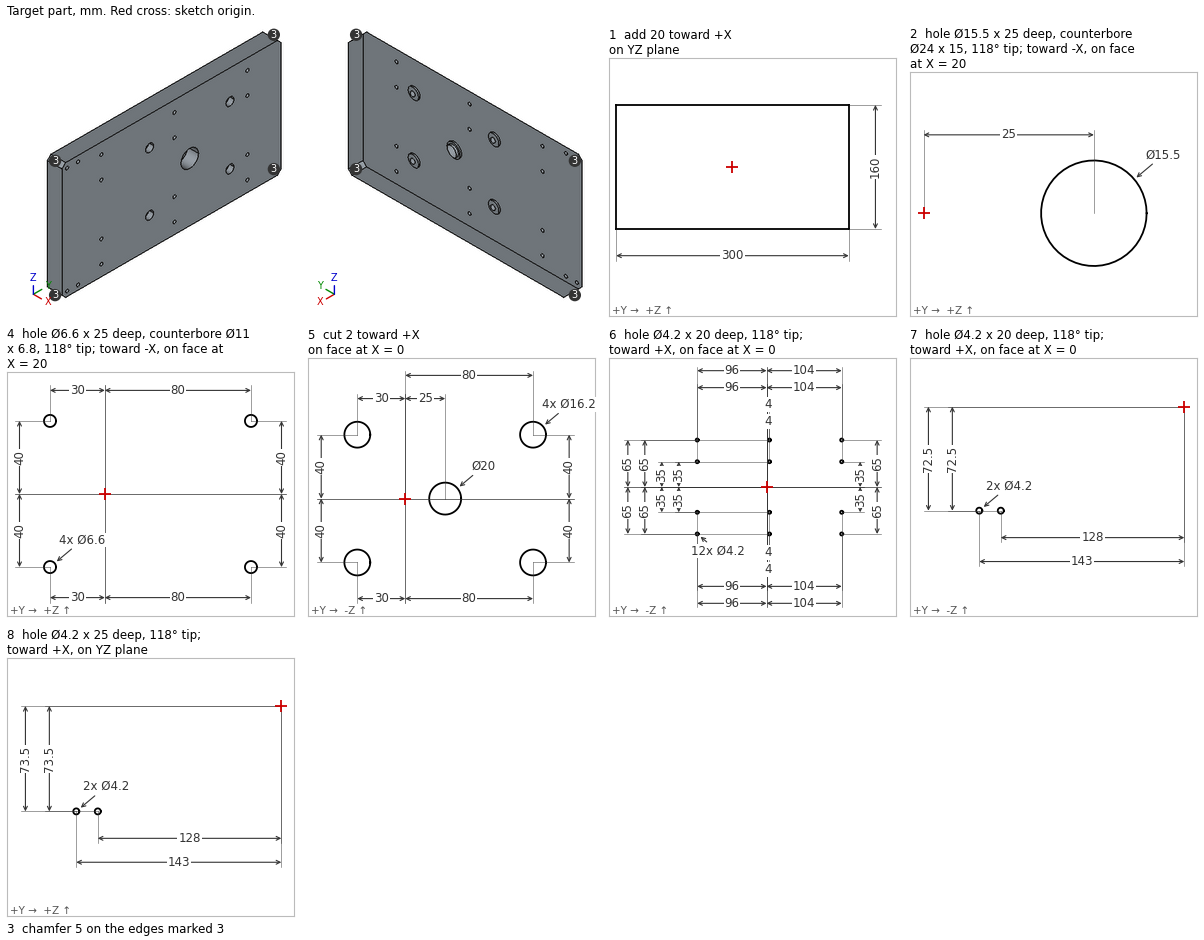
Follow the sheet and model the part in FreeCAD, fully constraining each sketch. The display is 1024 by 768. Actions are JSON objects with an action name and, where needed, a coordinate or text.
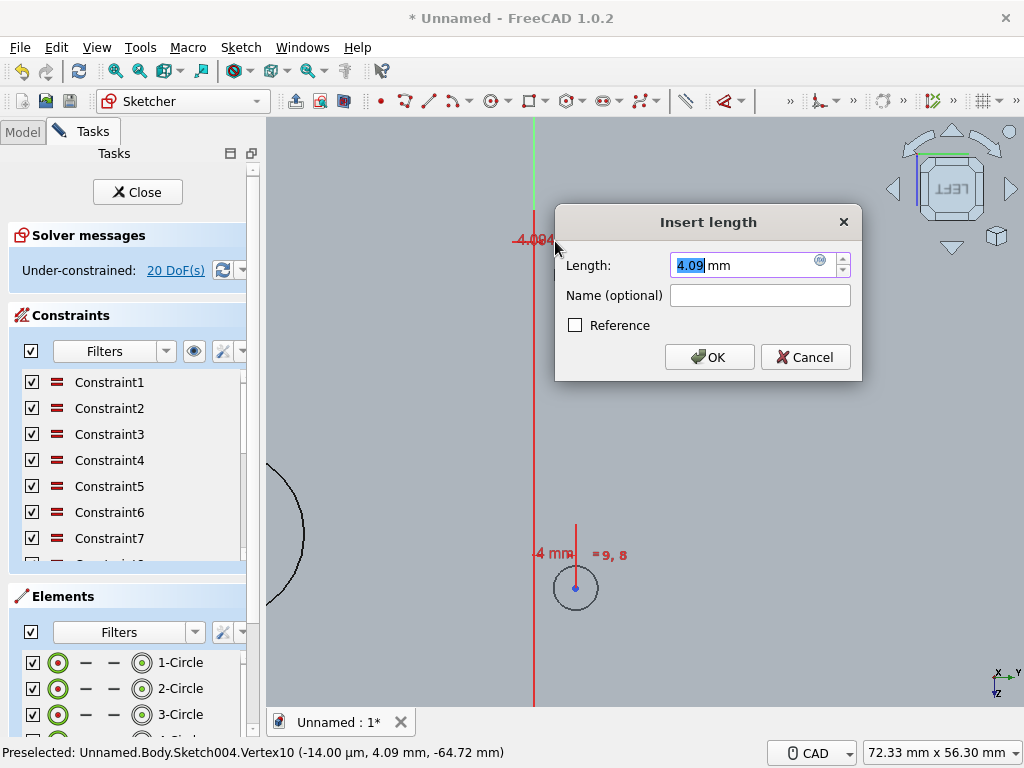
{"action": "type", "text": "4"}
{"action": "key", "text": "Return"}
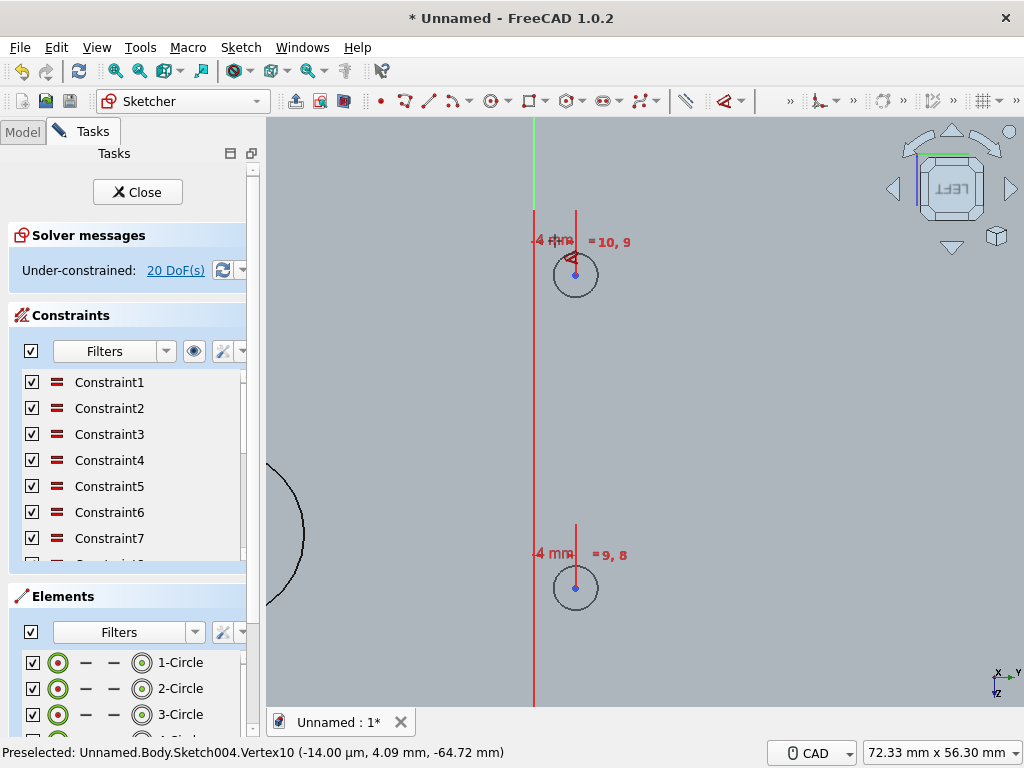
{"action": "scroll", "coordinate": [577, 275], "scroll_direction": "down", "scroll_amount": 8}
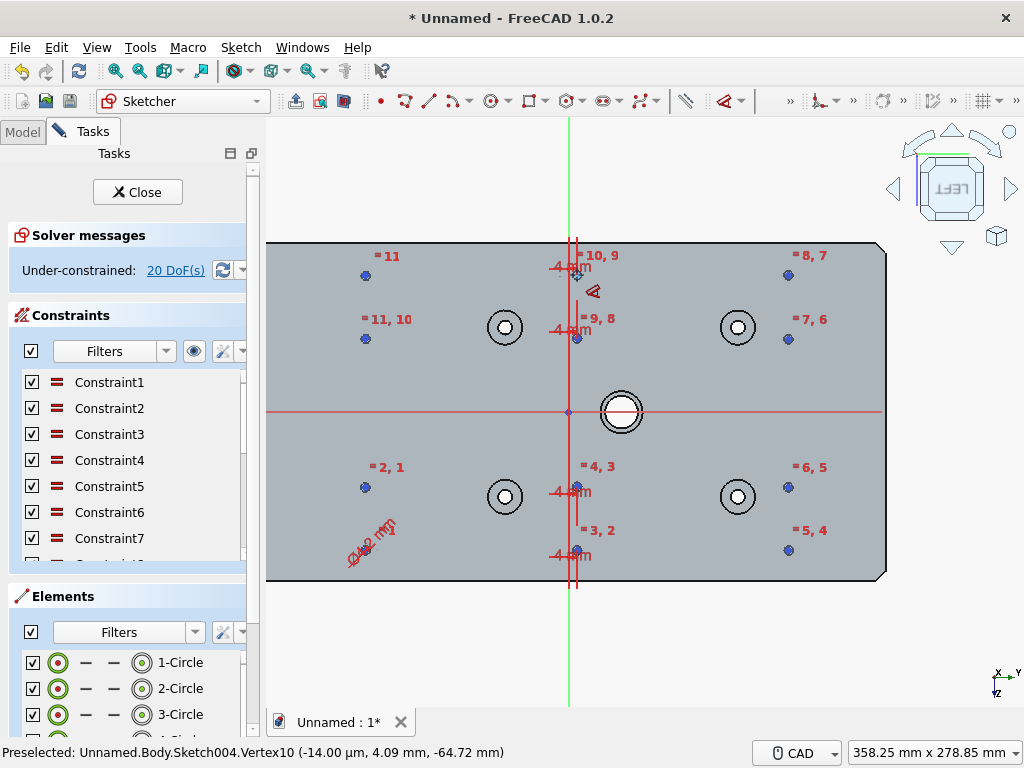
{"action": "left_click", "coordinate": [366, 550]}
{"action": "left_click", "coordinate": [467, 584]}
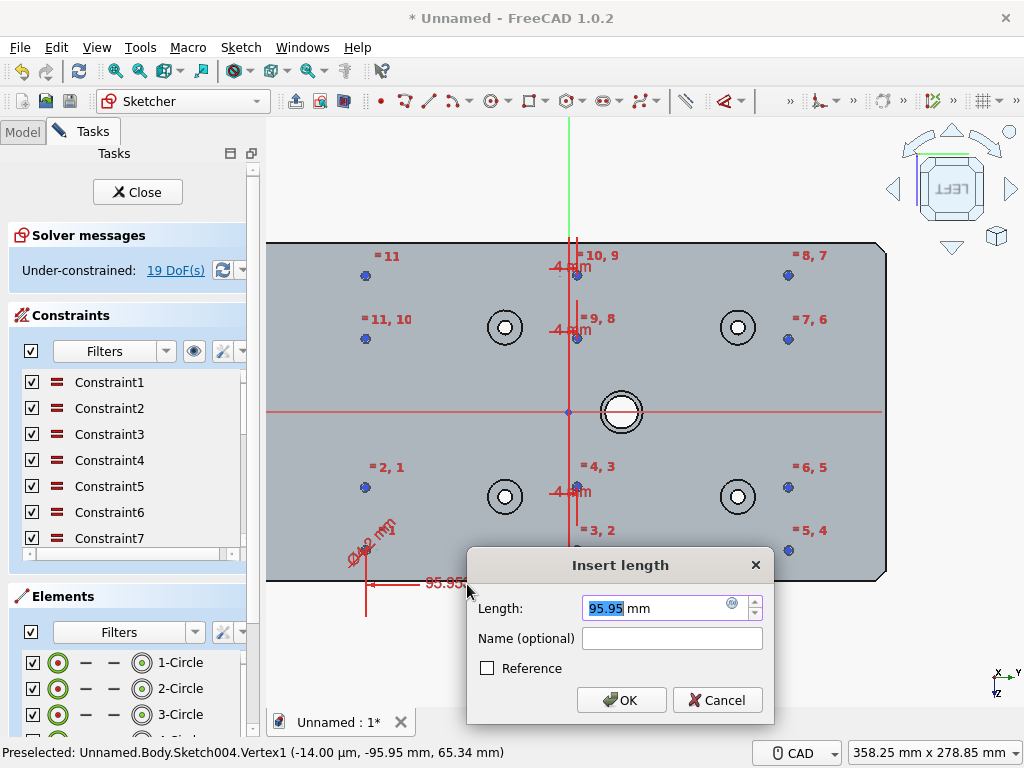
{"action": "type", "text": "96"}
{"action": "key", "text": "Return"}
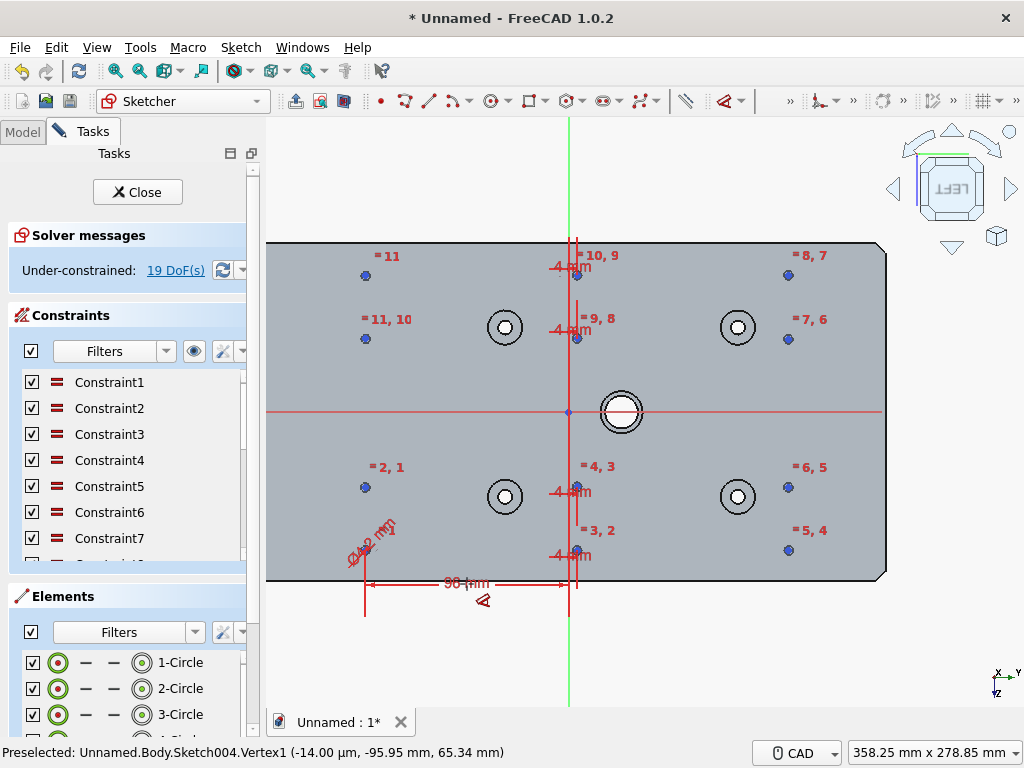
{"action": "left_click", "coordinate": [365, 550]}
{"action": "left_click", "coordinate": [331, 481]}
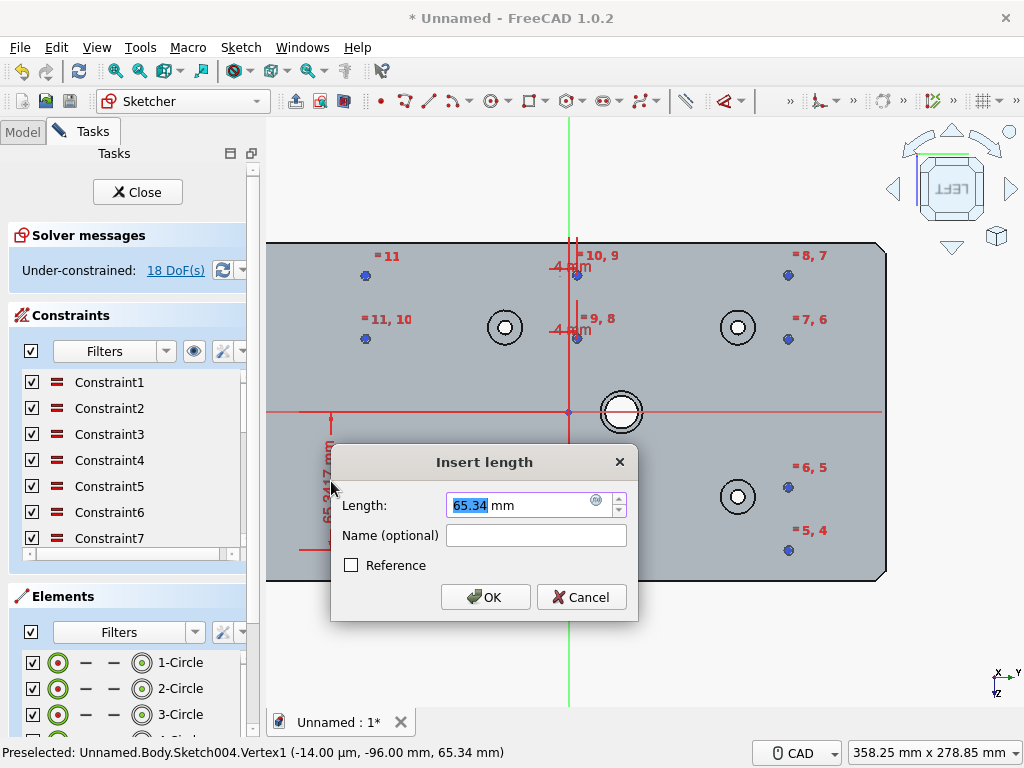
{"action": "type", "text": "65"}
{"action": "key", "text": "Return"}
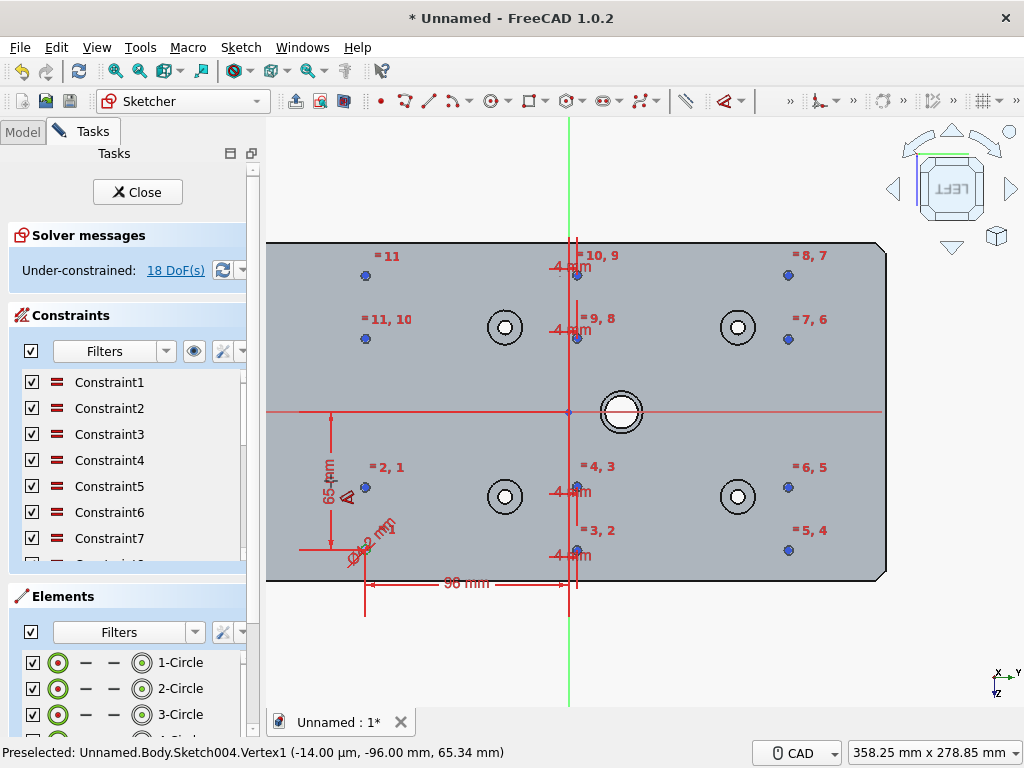
{"action": "left_click", "coordinate": [365, 487]}
{"action": "left_click", "coordinate": [467, 521]}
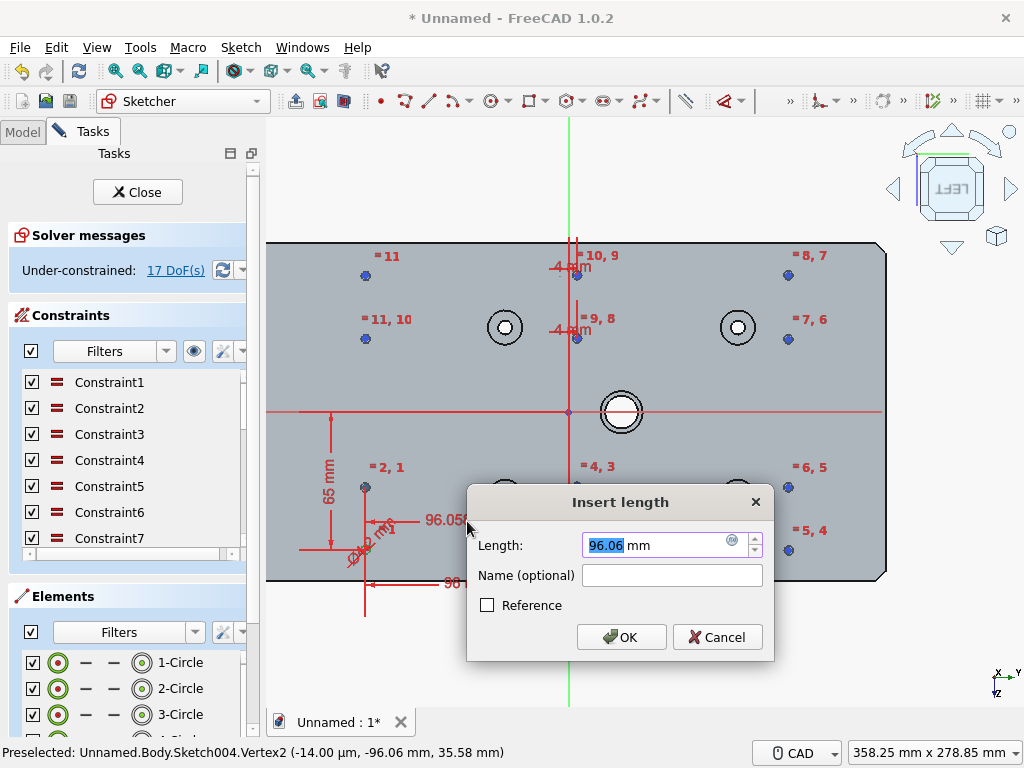
{"action": "type", "text": "96"}
{"action": "key", "text": "Return"}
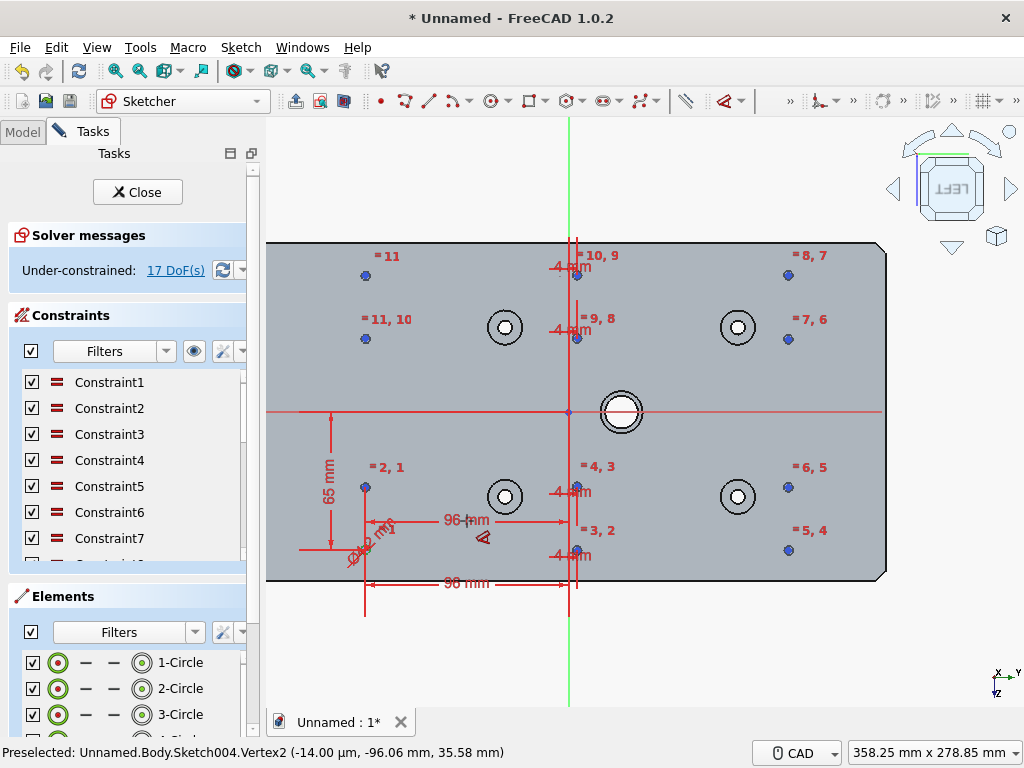
{"action": "left_click", "coordinate": [365, 487]}
{"action": "left_click", "coordinate": [331, 450]}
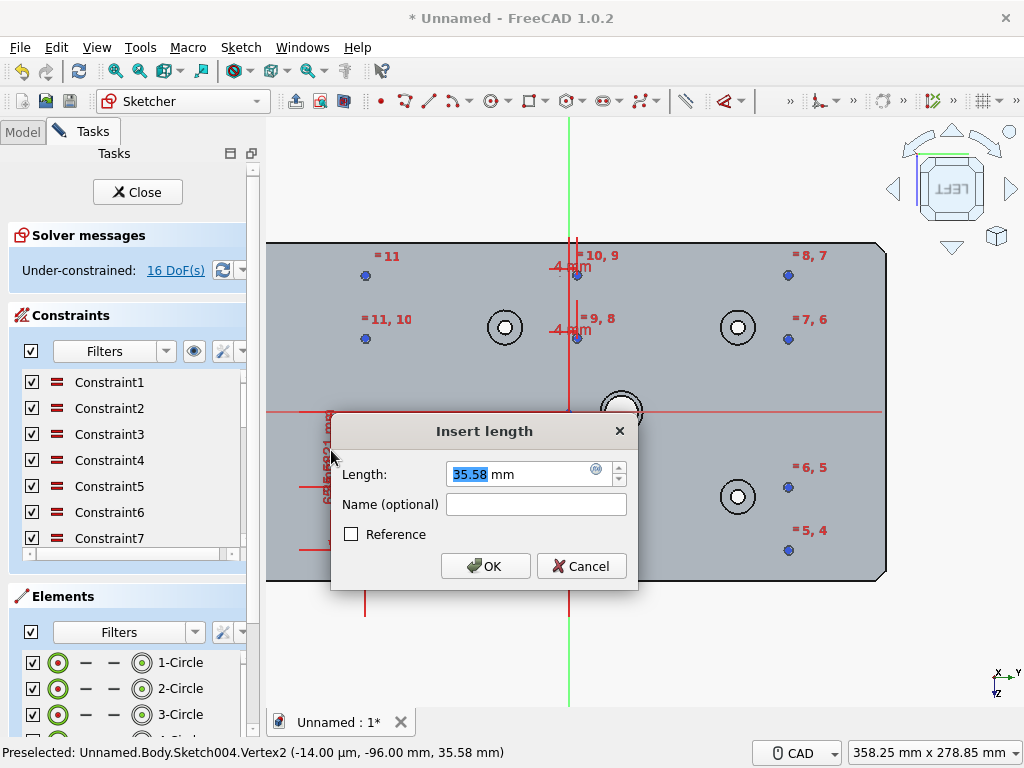
{"action": "type", "text": "35"}
{"action": "key", "text": "Return"}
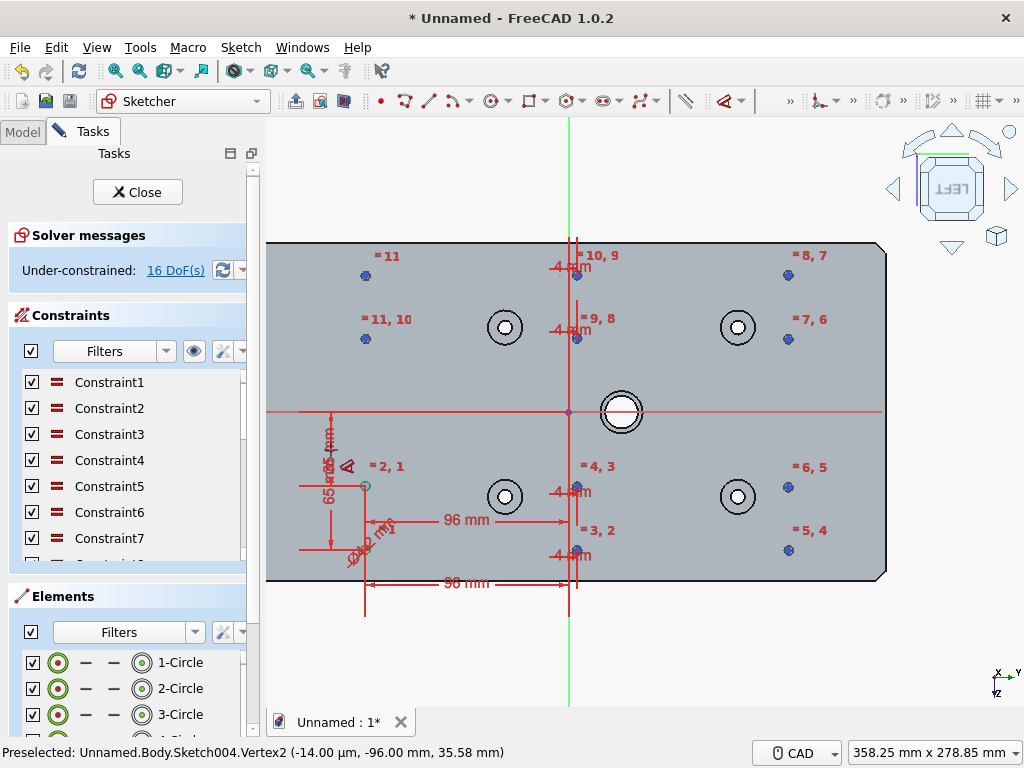
{"action": "left_click", "coordinate": [577, 550]}
{"action": "left_click", "coordinate": [535, 449]}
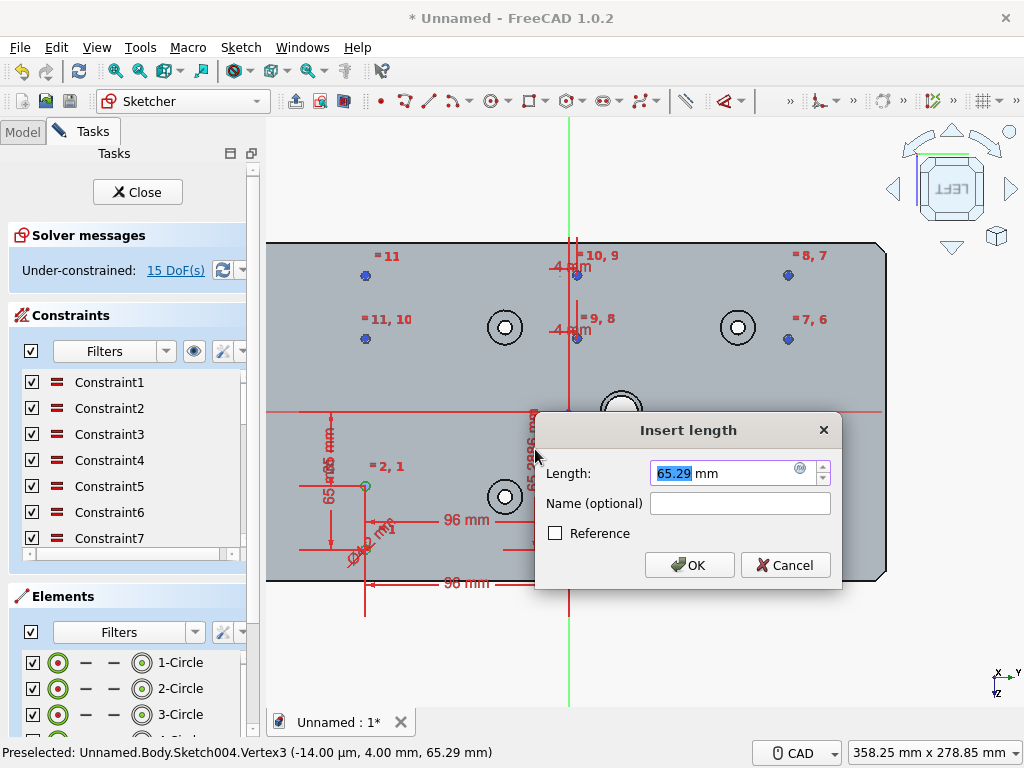
{"action": "type", "text": "65"}
{"action": "key", "text": "Return"}